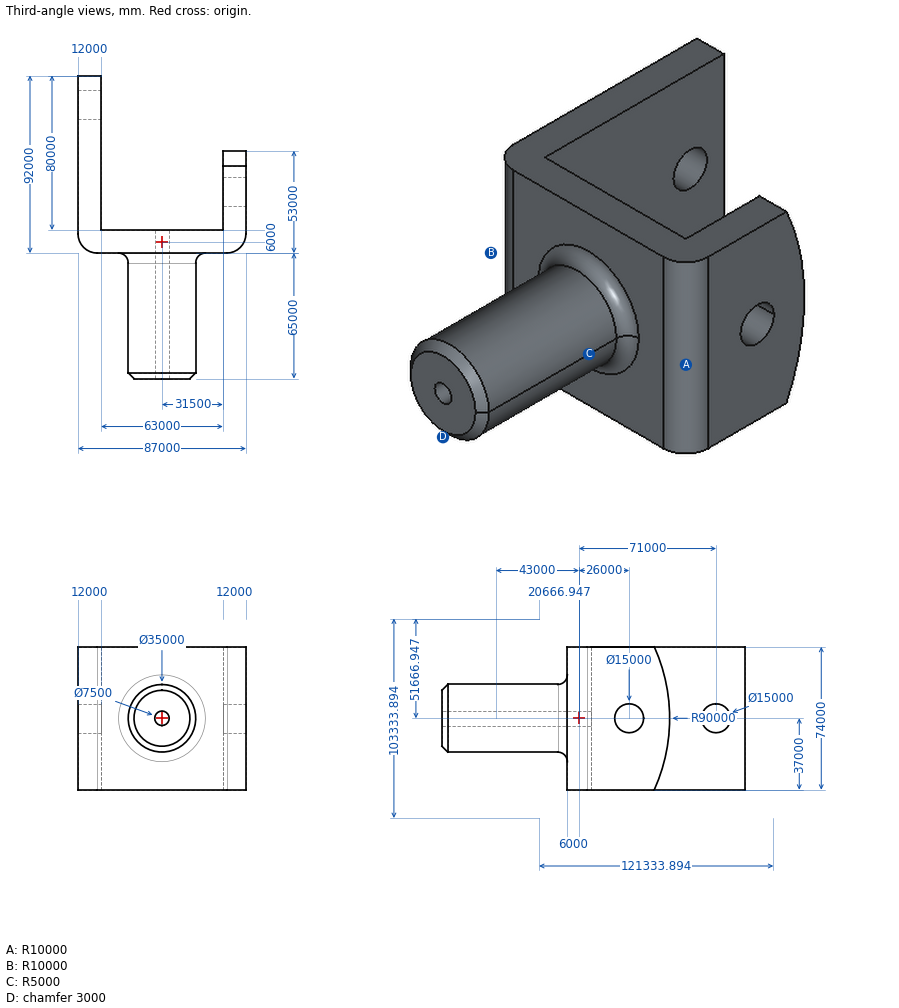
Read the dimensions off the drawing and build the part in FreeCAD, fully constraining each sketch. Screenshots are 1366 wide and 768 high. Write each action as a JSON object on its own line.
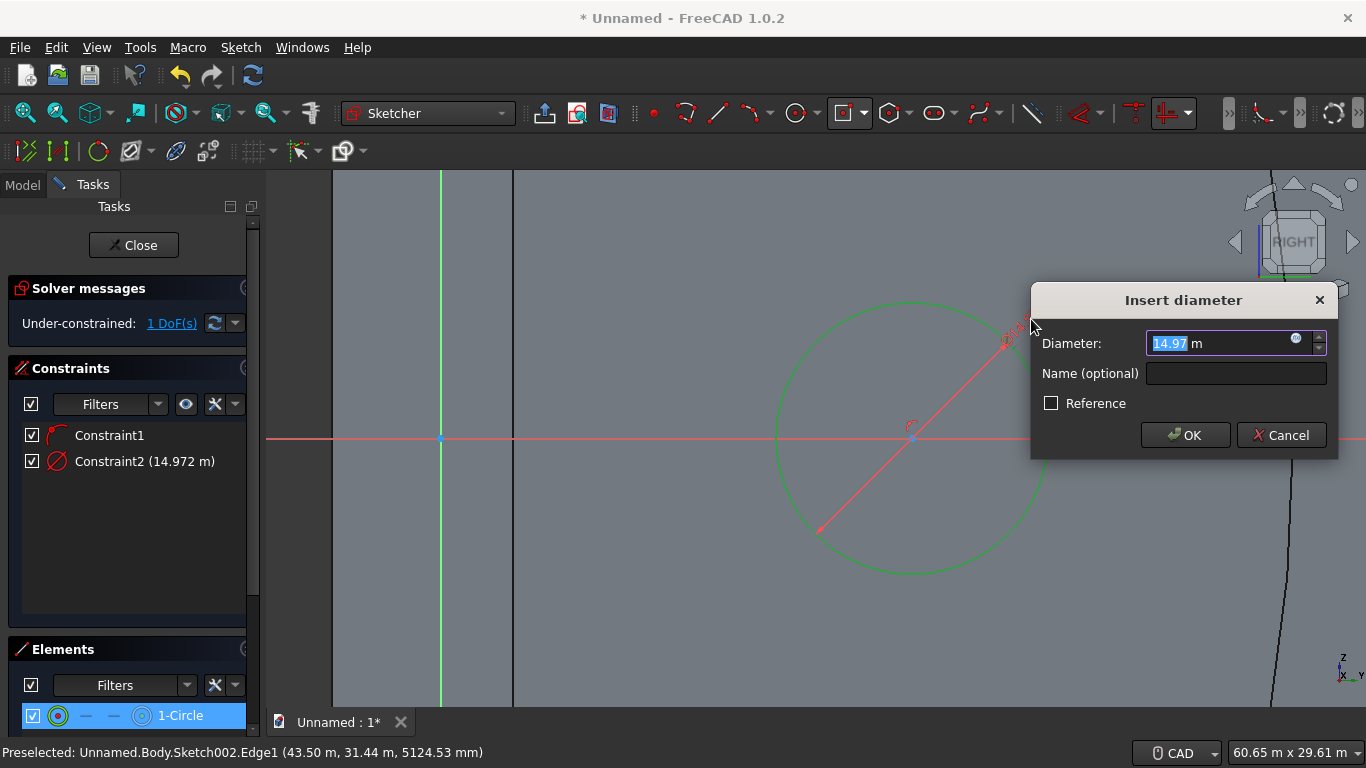
{"action": "key", "text": "ctrl+a"}
{"action": "type", "text": "15000 mm"}
{"action": "key", "text": "Return"}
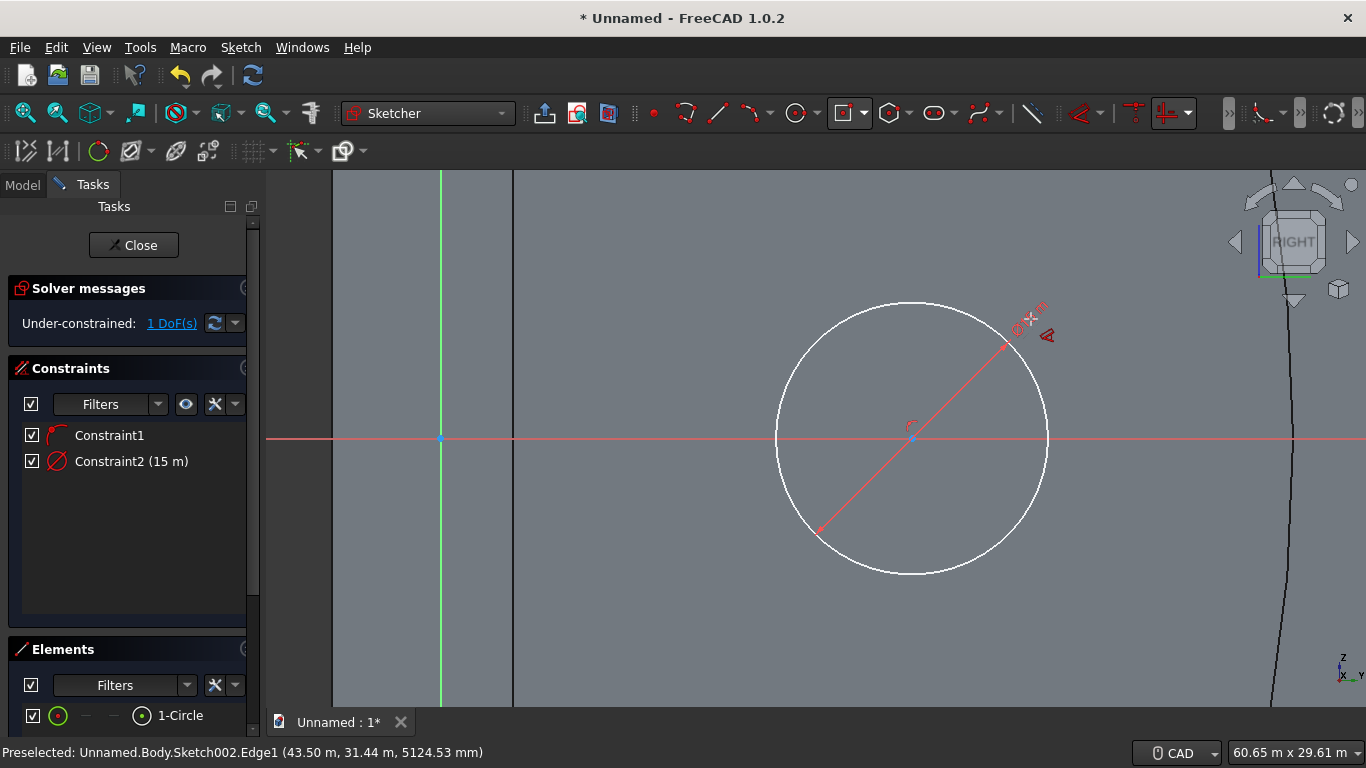
{"action": "left_click", "coordinate": [912, 438]}
{"action": "left_click", "coordinate": [676, 472]}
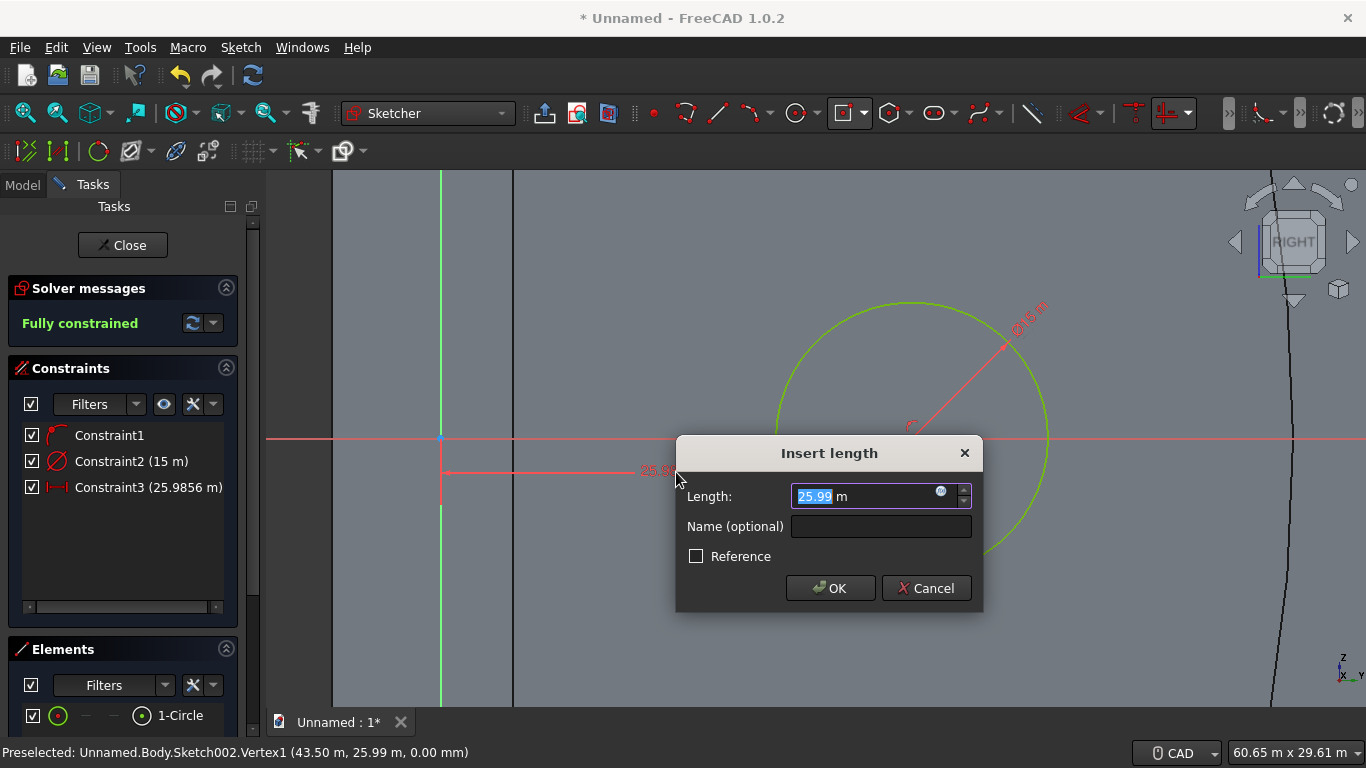
{"action": "key", "text": "ctrl+a"}
{"action": "type", "text": "26000 mm"}
{"action": "key", "text": "Return"}
{"action": "key", "text": "Escape"}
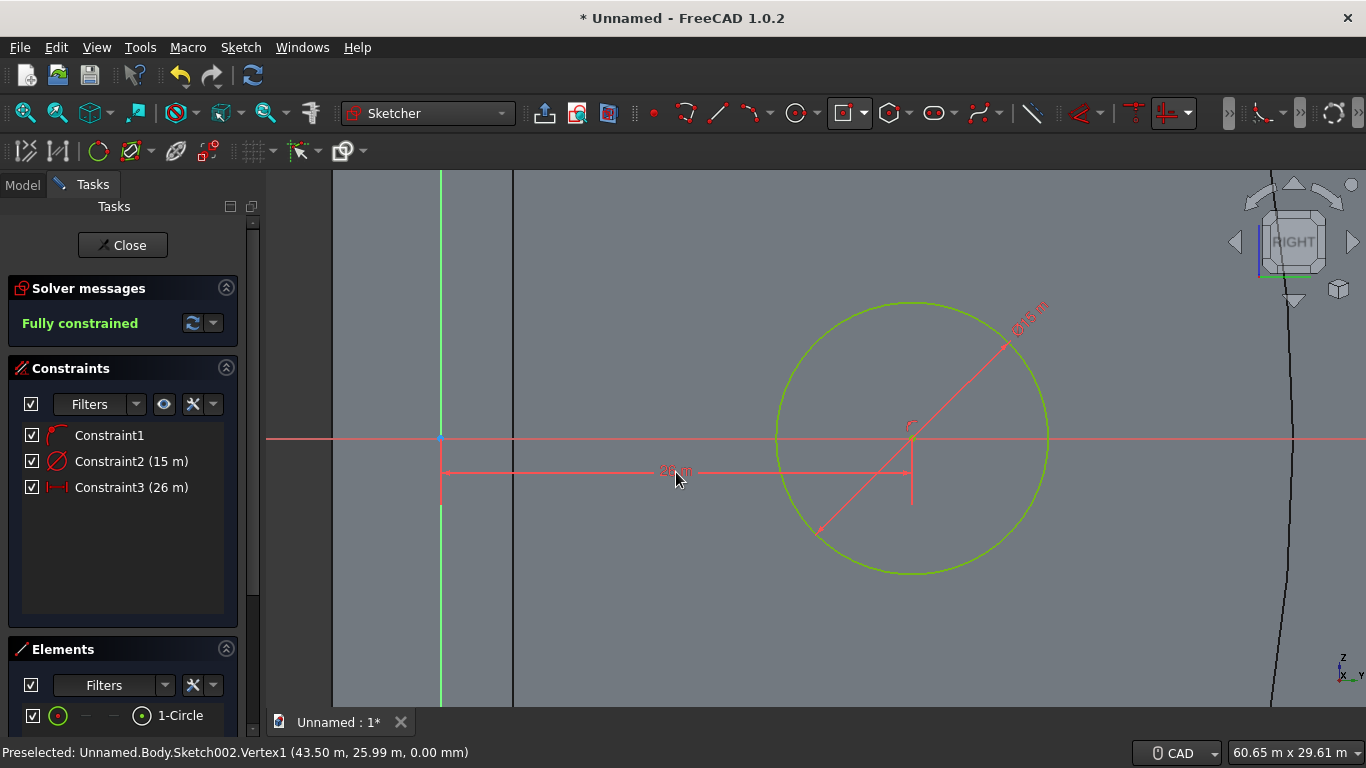
{"action": "left_click", "coordinate": [123, 245]}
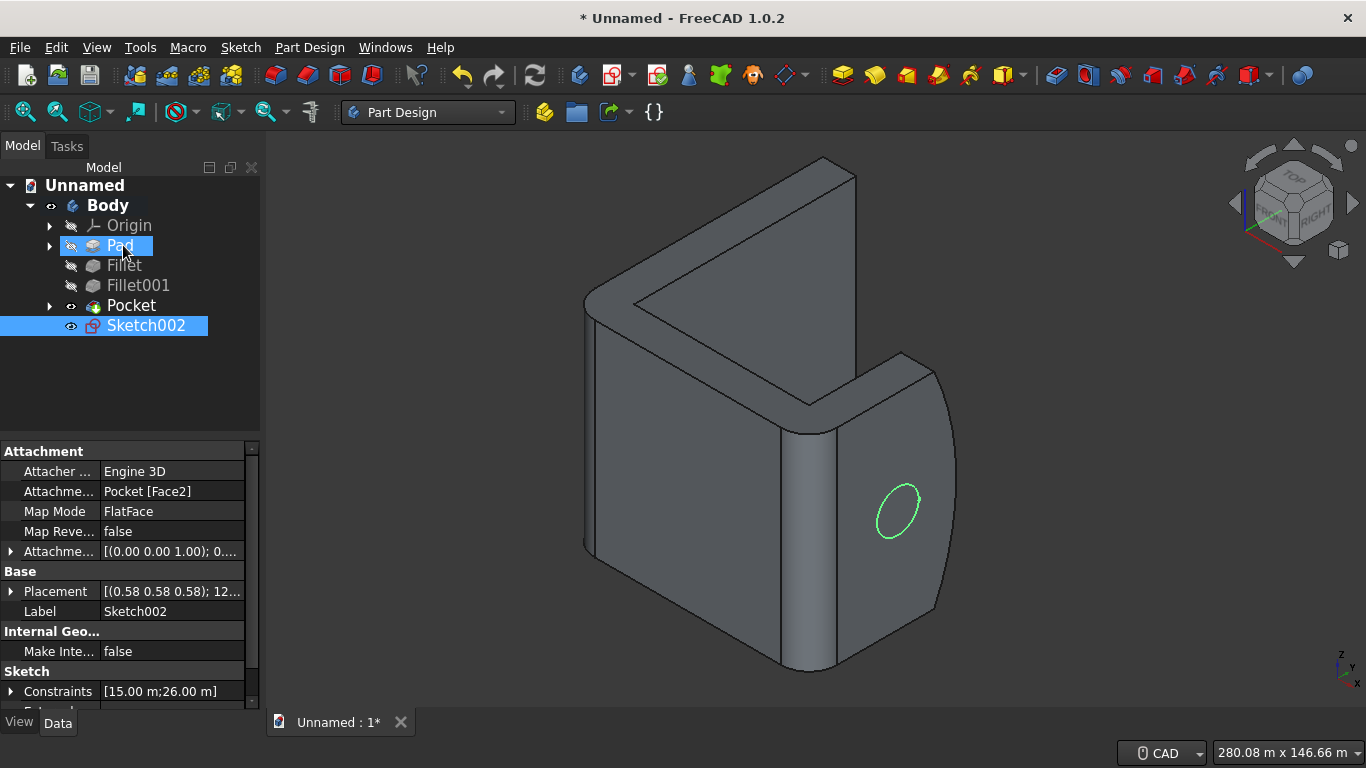
{"action": "left_click", "coordinate": [1058, 76]}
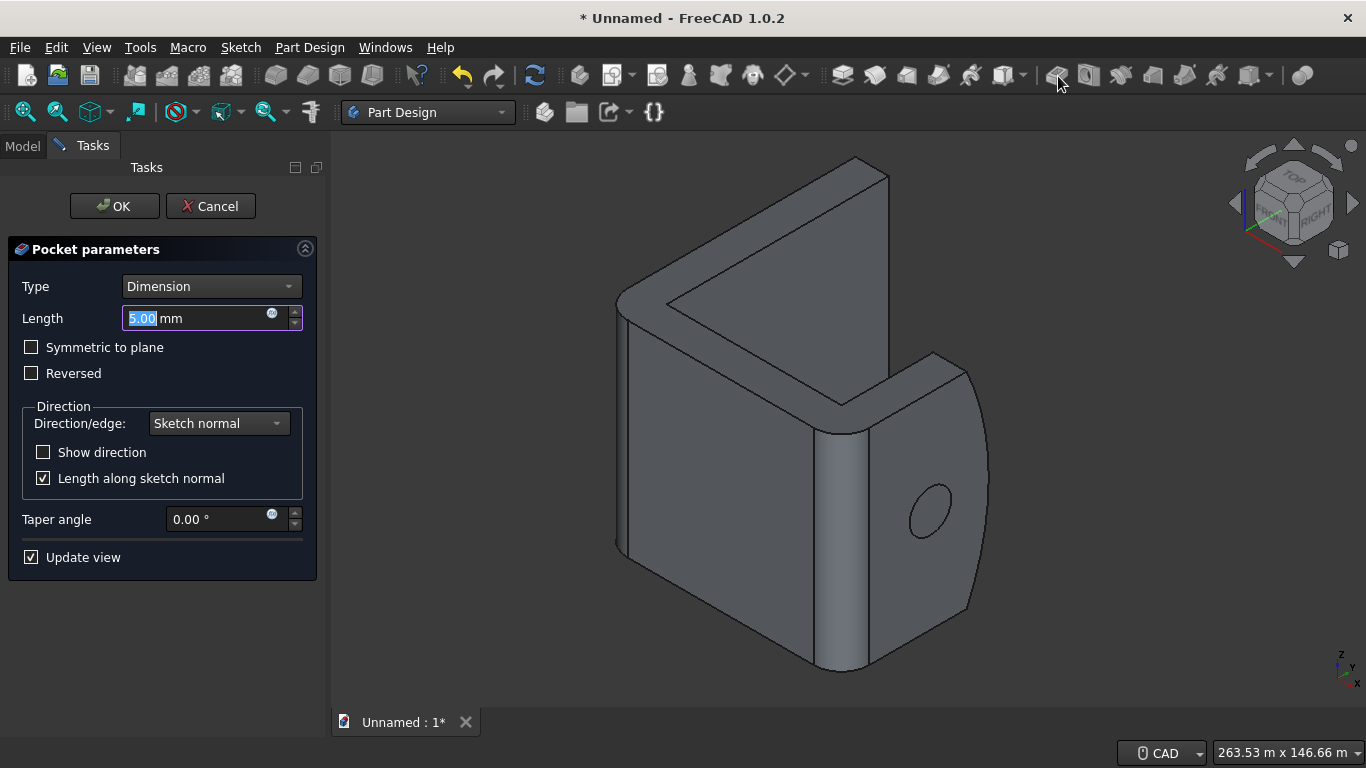
{"action": "type", "text": "12000"}
{"action": "key", "text": "Tab"}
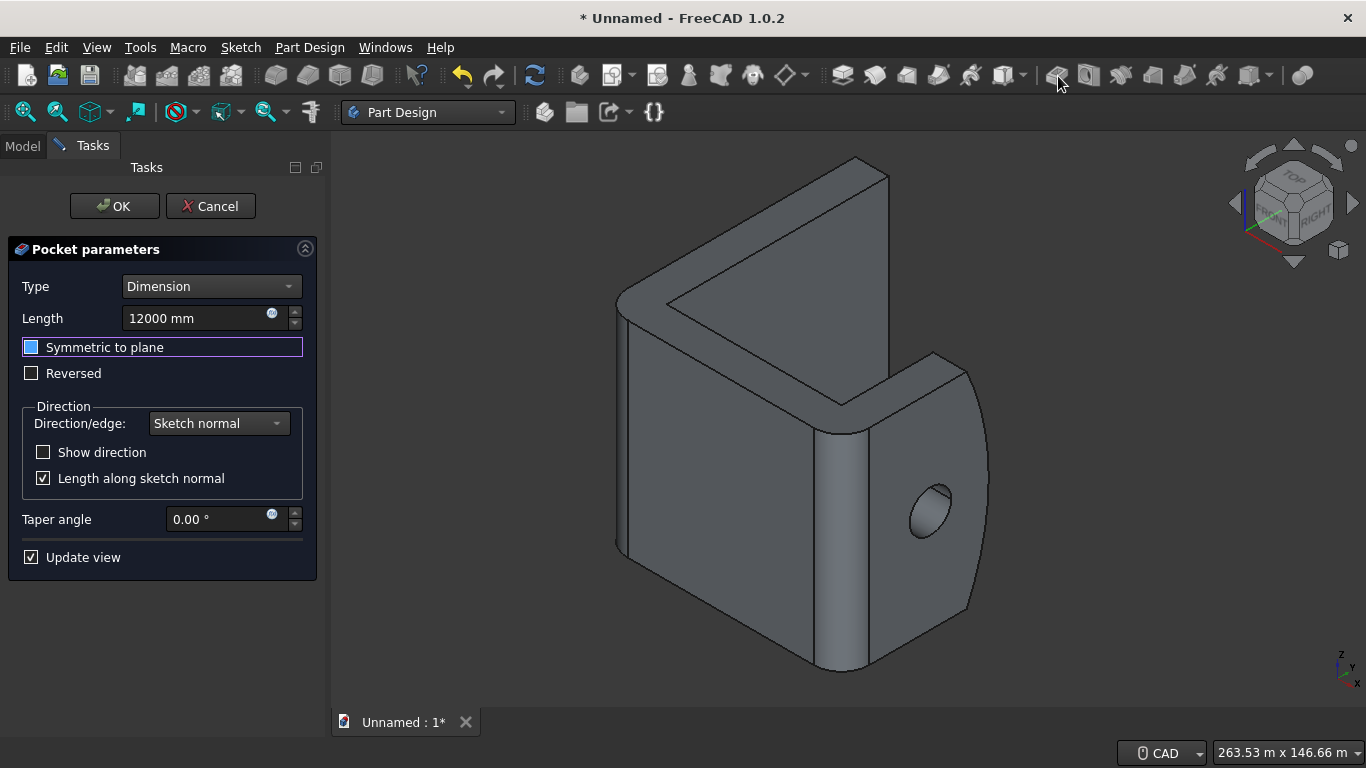
{"action": "left_click", "coordinate": [115, 206]}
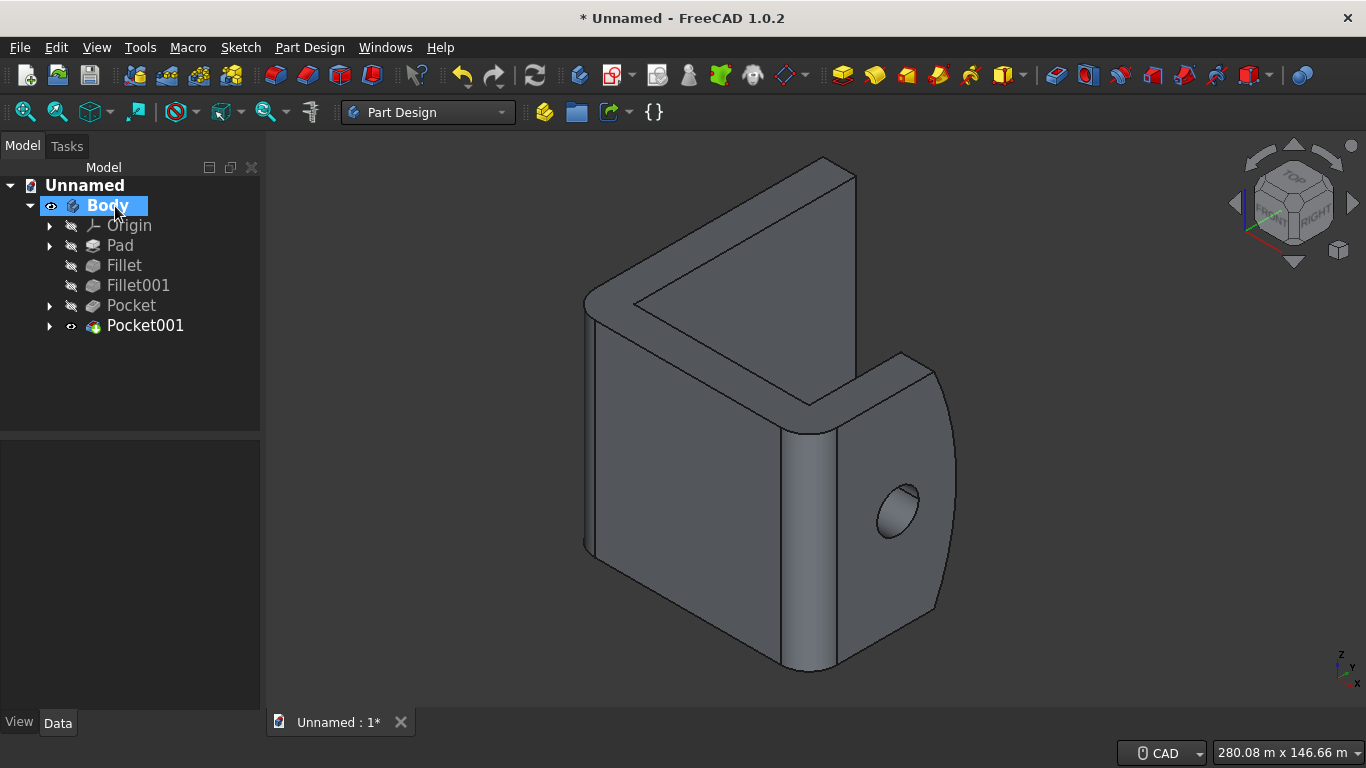
{"action": "key", "text": "6"}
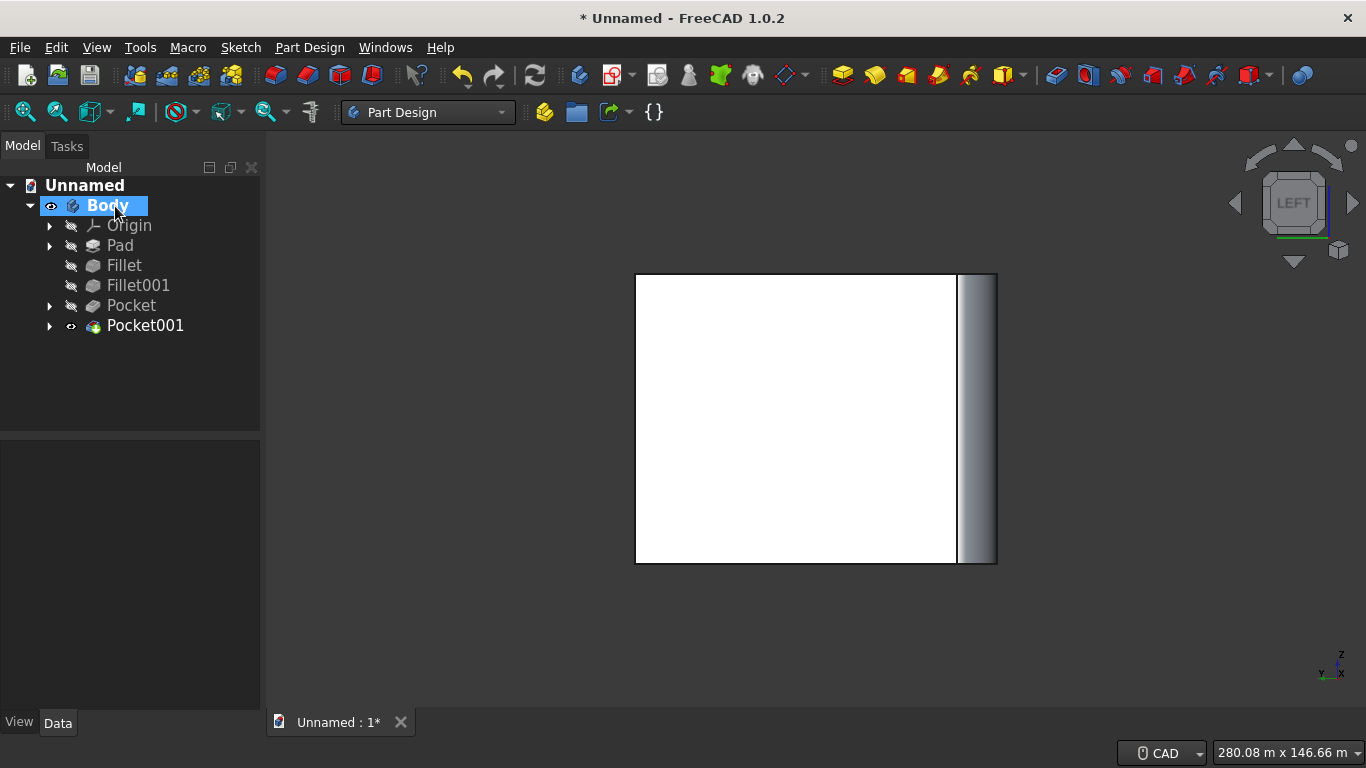
{"action": "left_click", "coordinate": [796, 418]}